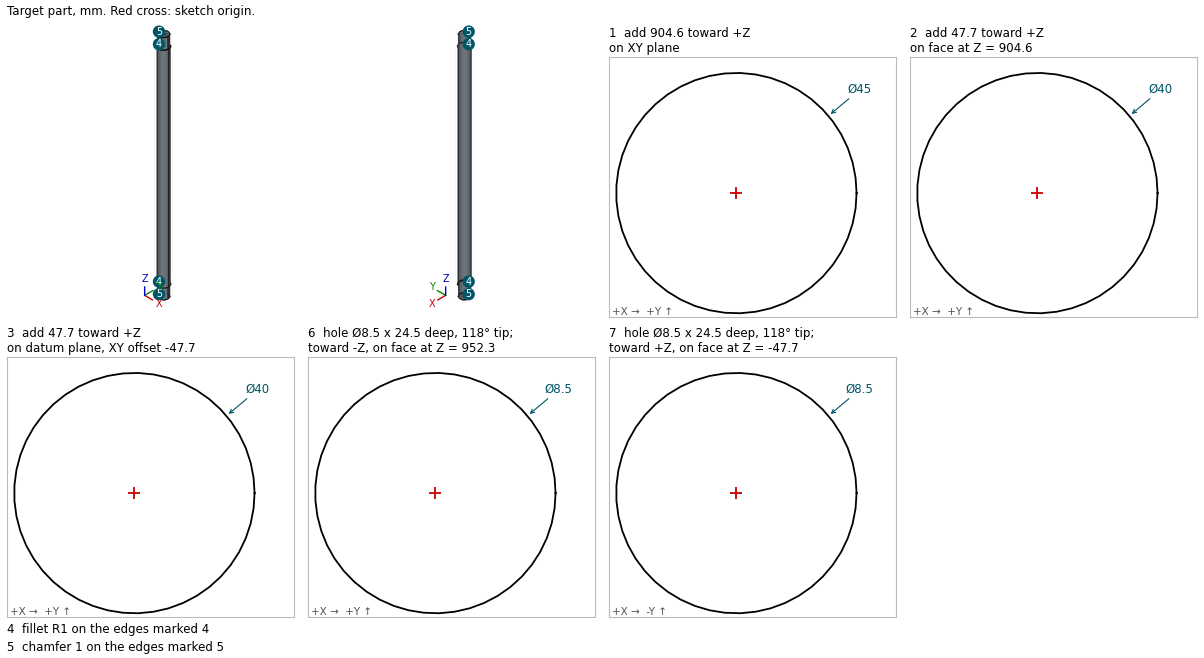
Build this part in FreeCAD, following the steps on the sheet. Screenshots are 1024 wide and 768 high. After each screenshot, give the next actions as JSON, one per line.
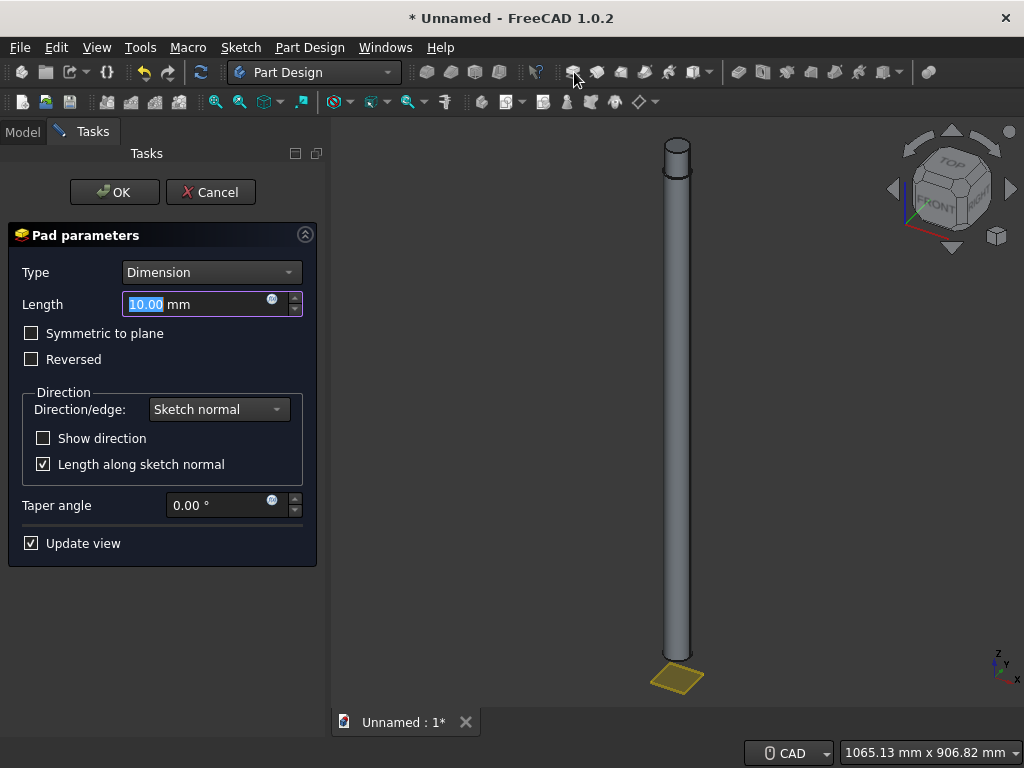
{"action": "type", "text": "47.7"}
{"action": "key", "text": "Tab"}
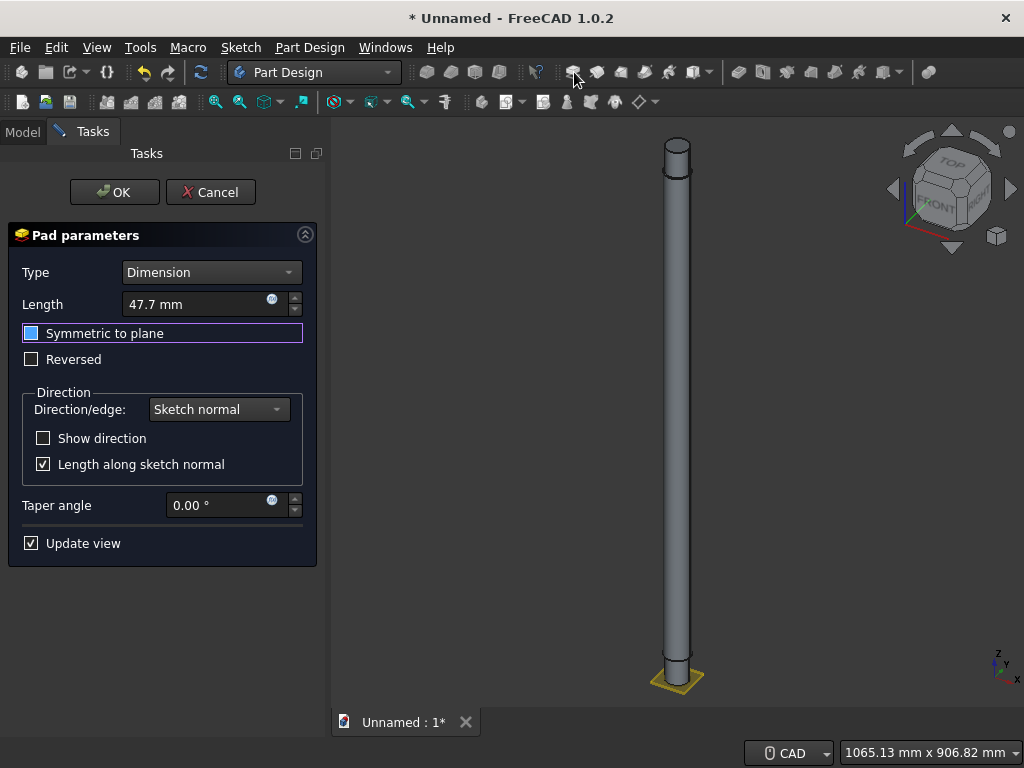
{"action": "left_click", "coordinate": [115, 192]}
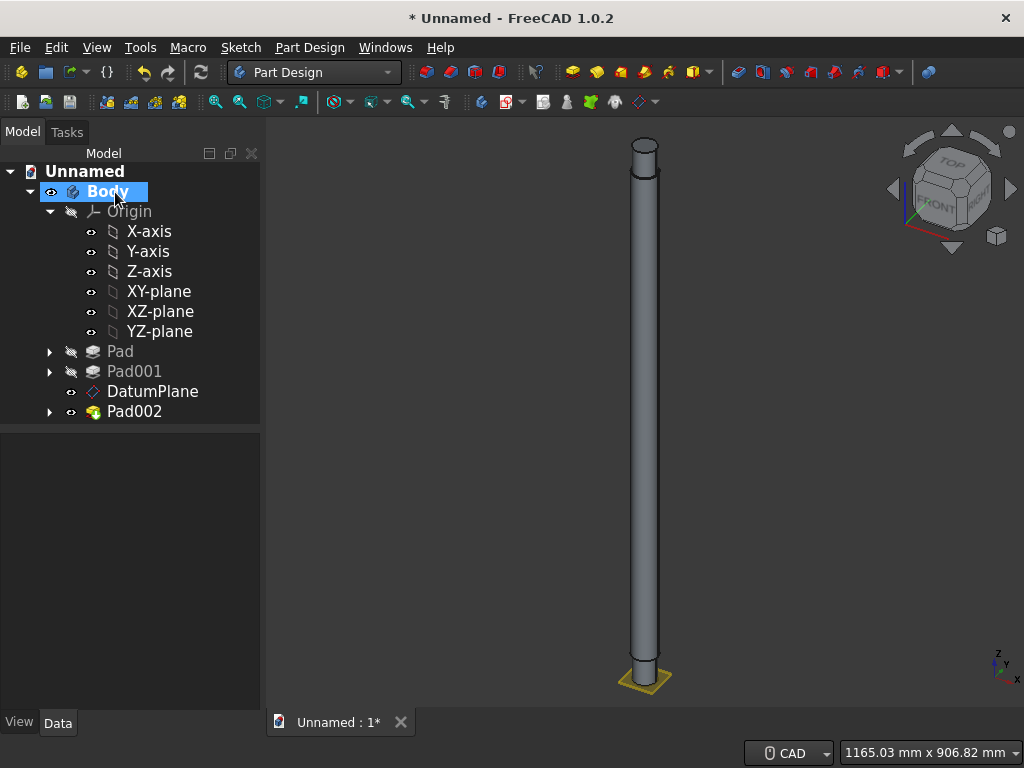
{"action": "left_click", "coordinate": [116, 392]}
{"action": "key", "text": "space"}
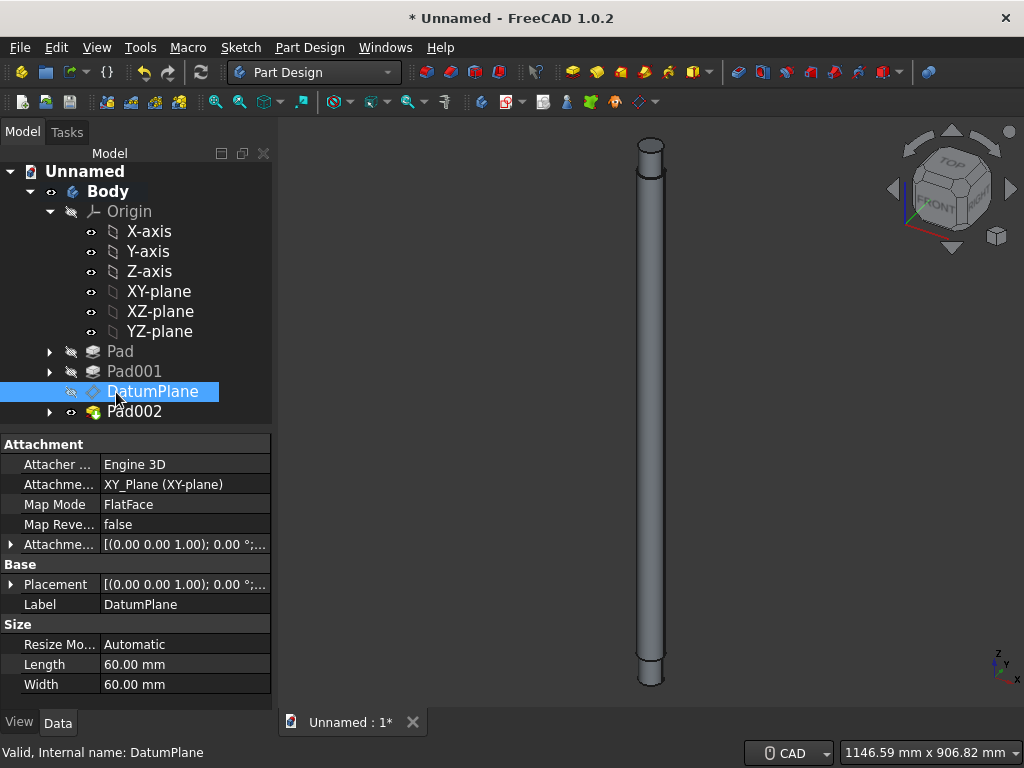
{"action": "key", "text": "0"}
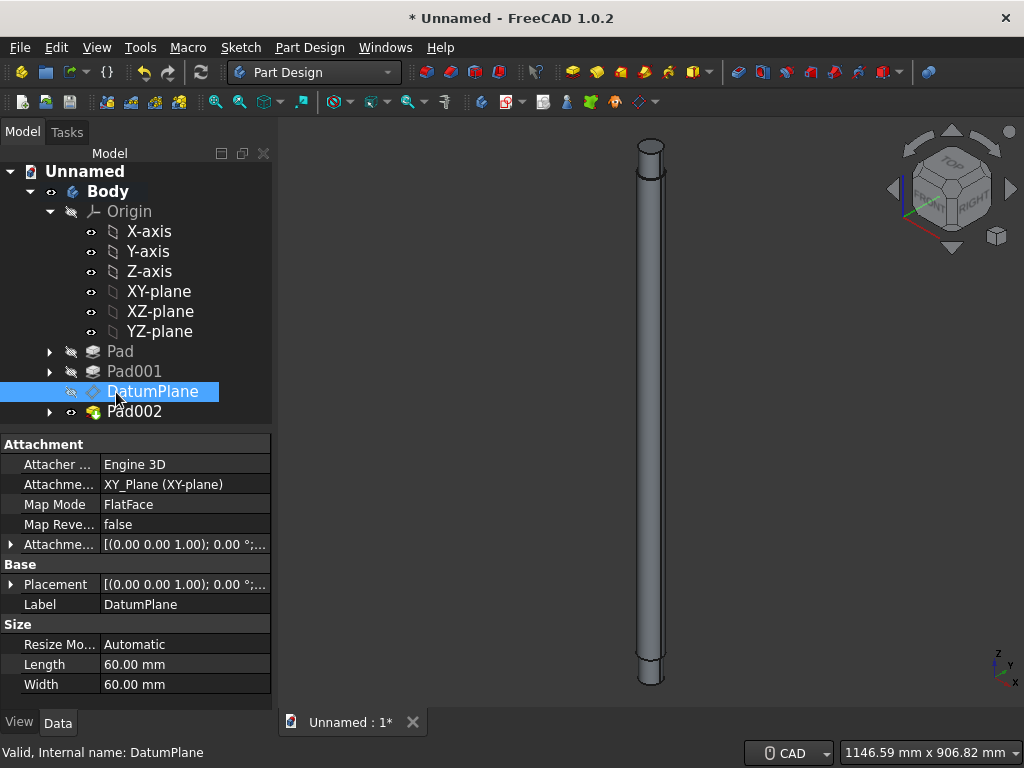
{"action": "key", "text": "2"}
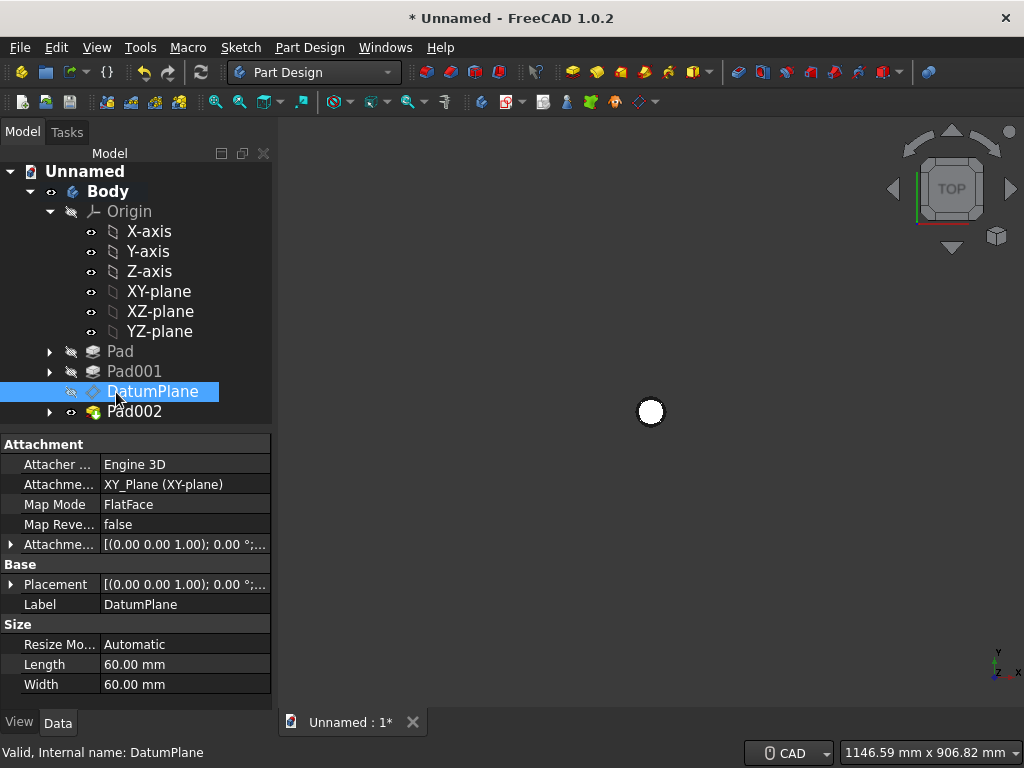
{"action": "left_click", "coordinate": [216, 102]}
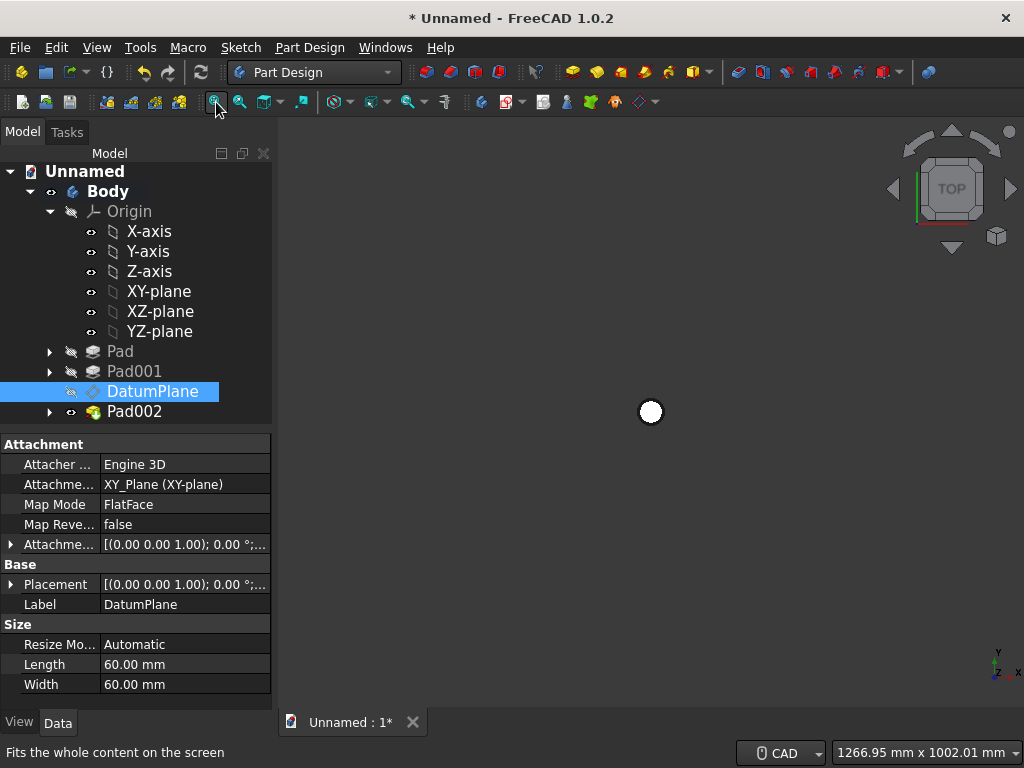
{"action": "key", "text": "1"}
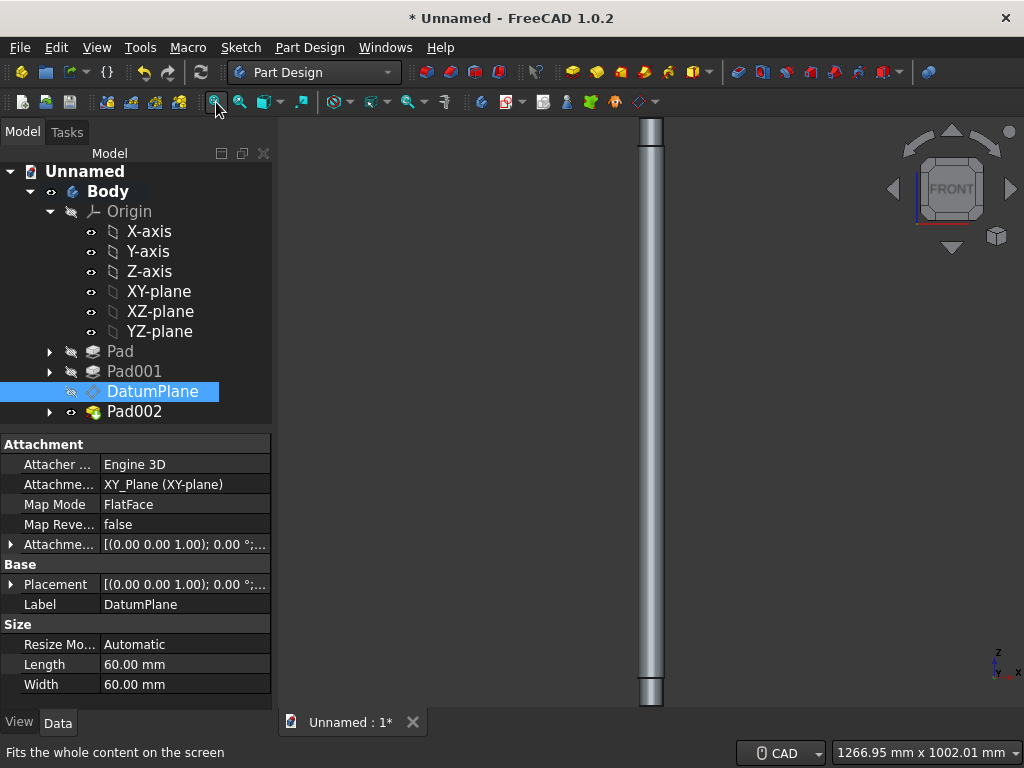
{"action": "key", "text": "3"}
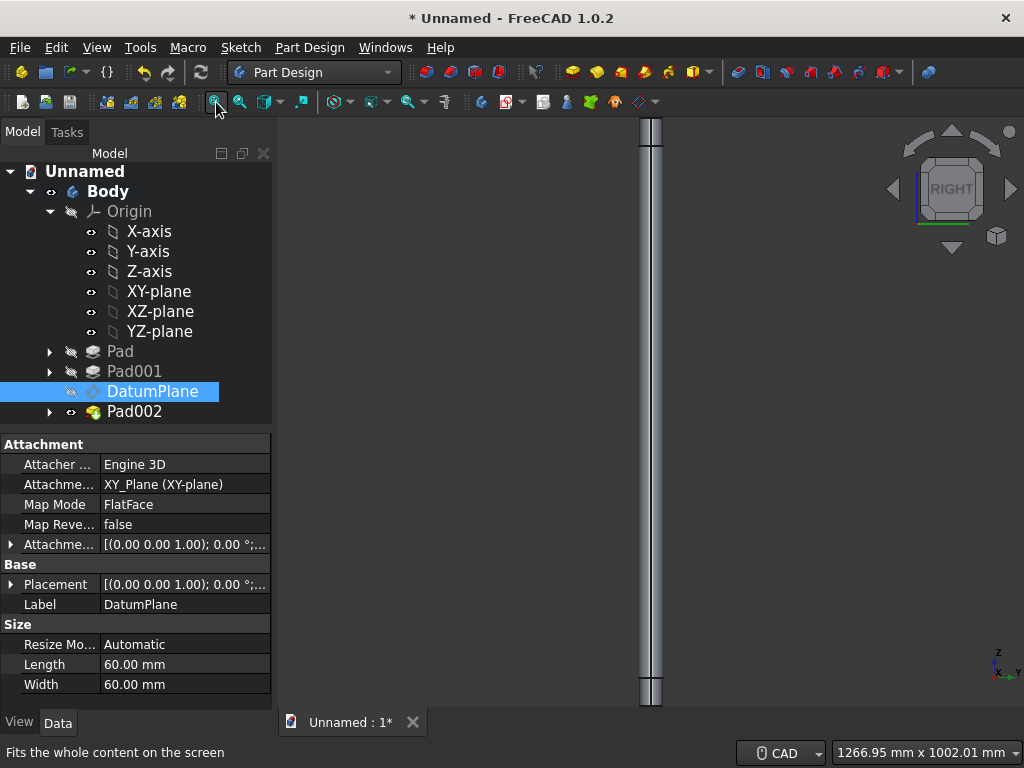
{"action": "key", "text": "5"}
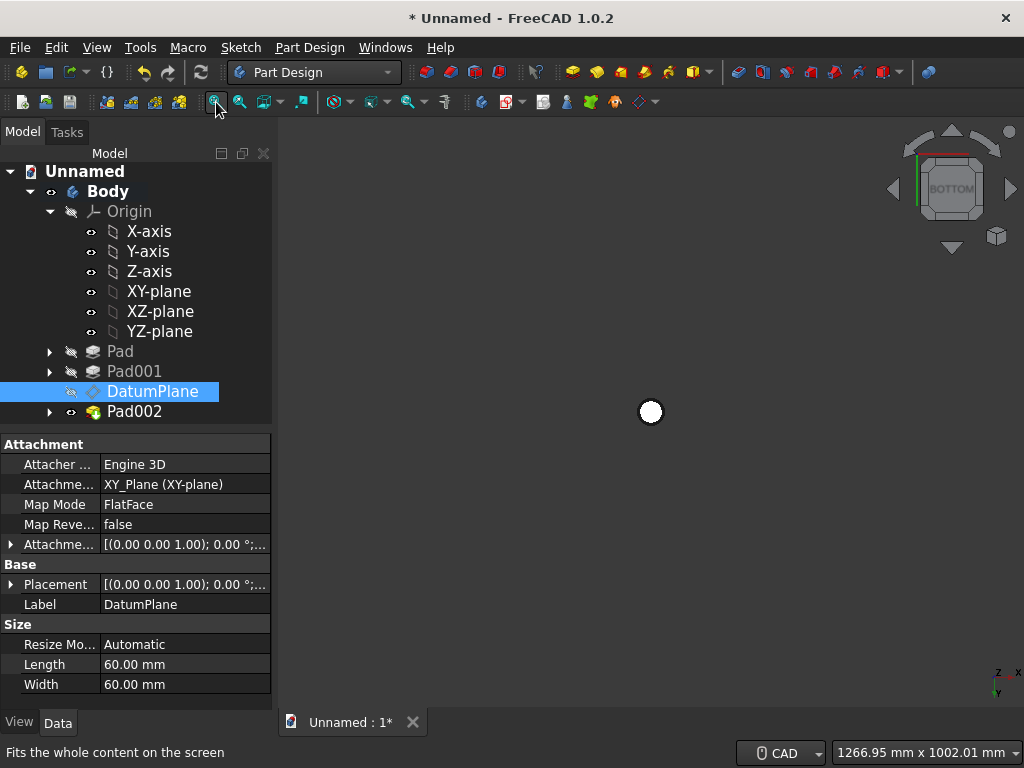
{"action": "key", "text": "v f"}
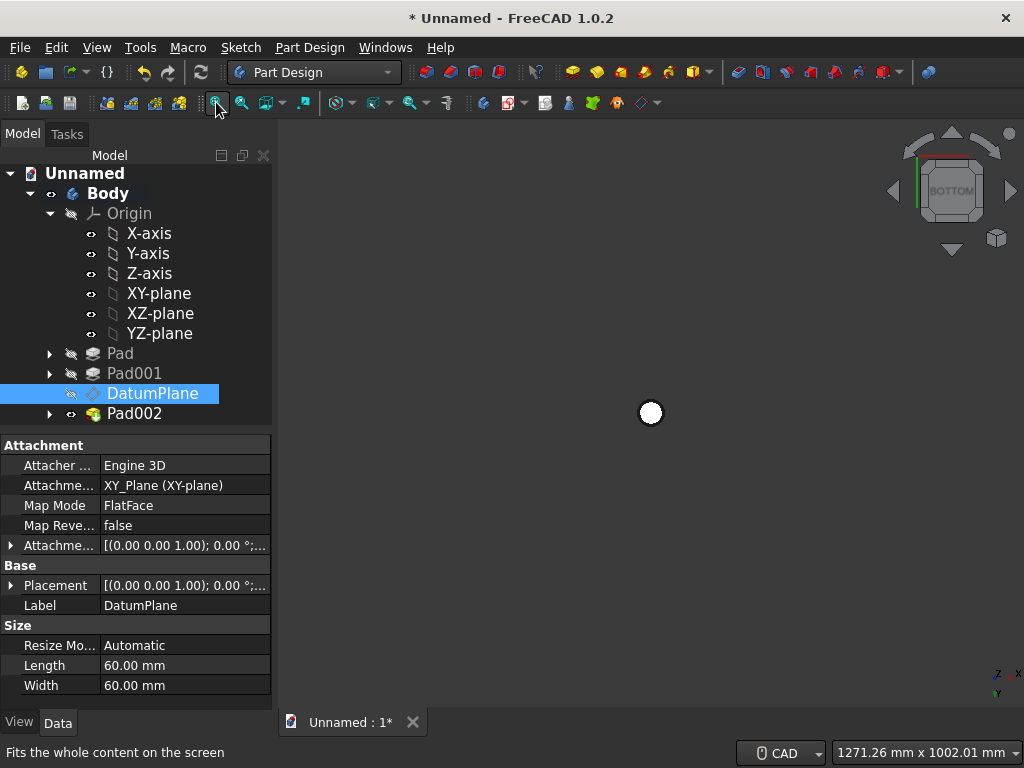
{"action": "key", "text": "4"}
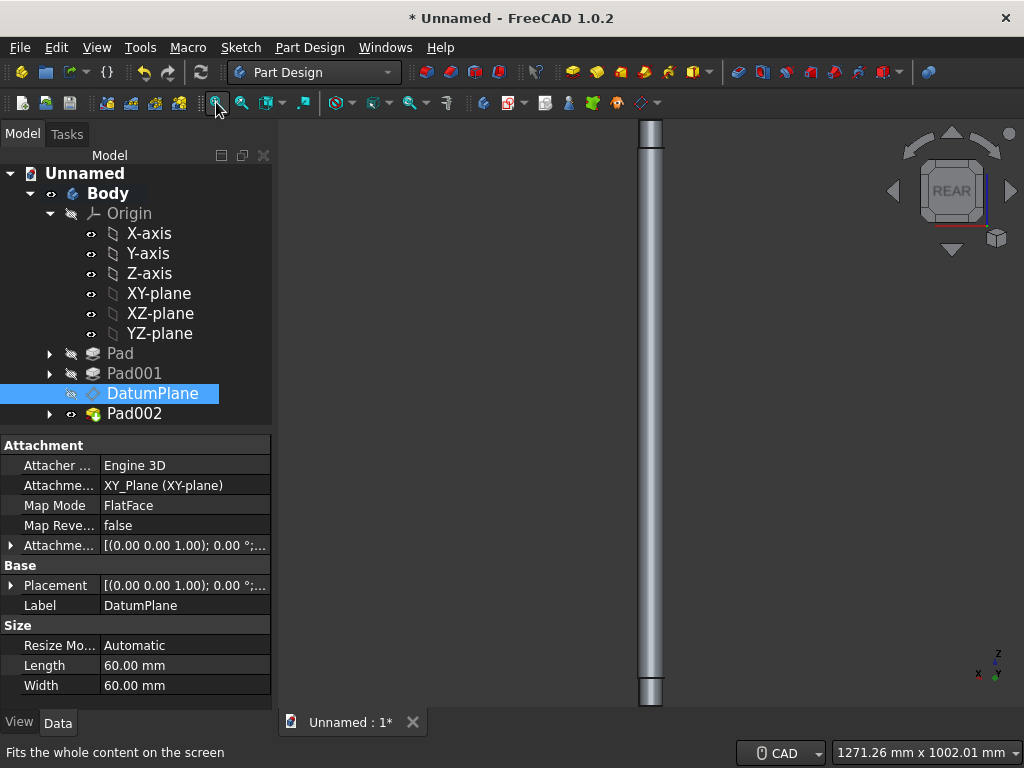
{"action": "key", "text": "6"}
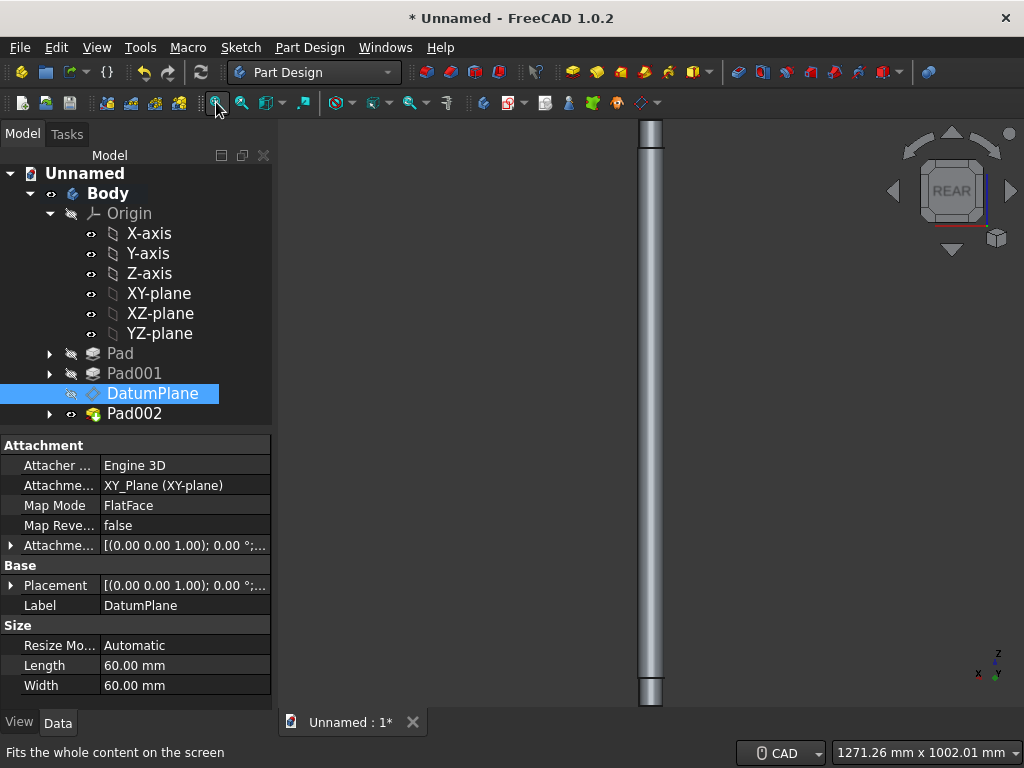
{"action": "key", "text": "v 3"}